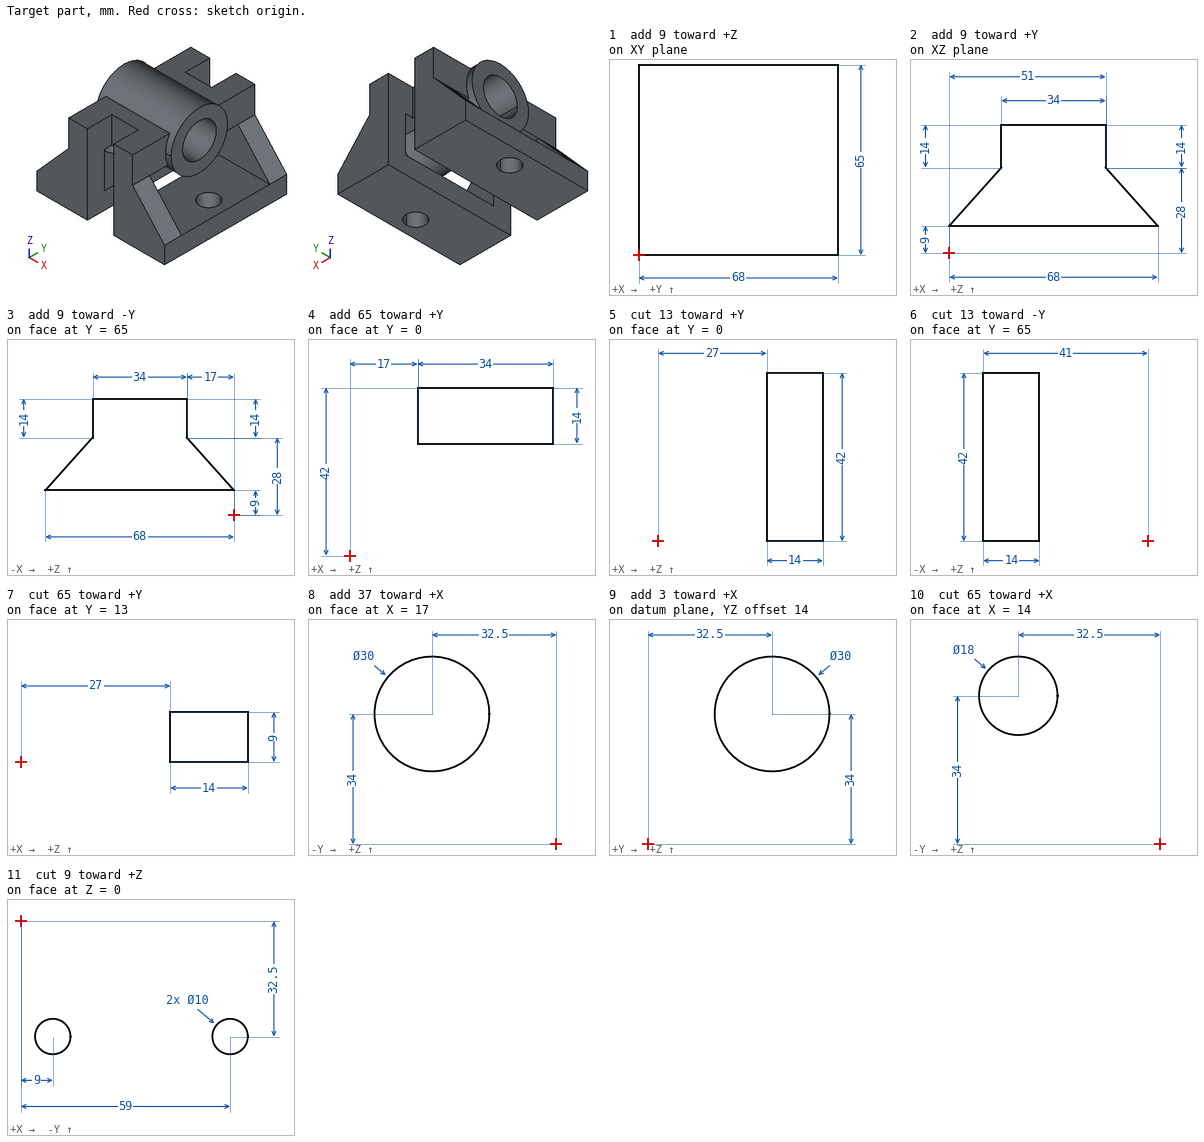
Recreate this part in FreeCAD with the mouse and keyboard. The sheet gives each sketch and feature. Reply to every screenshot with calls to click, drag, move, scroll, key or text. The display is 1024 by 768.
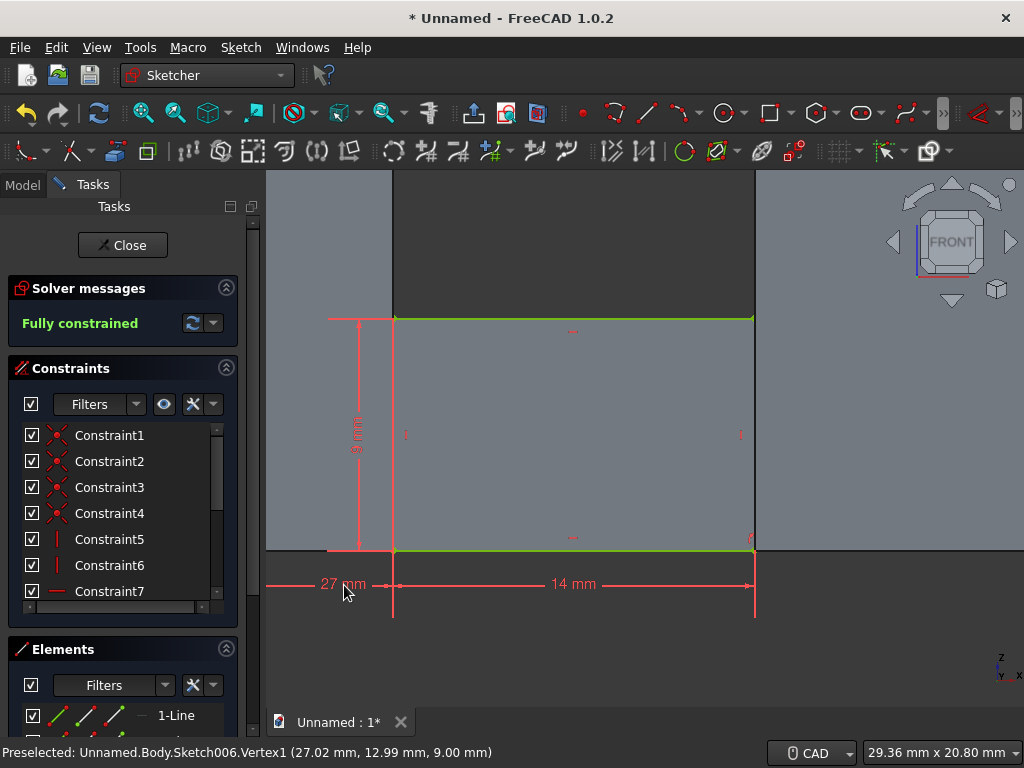
click(123, 245)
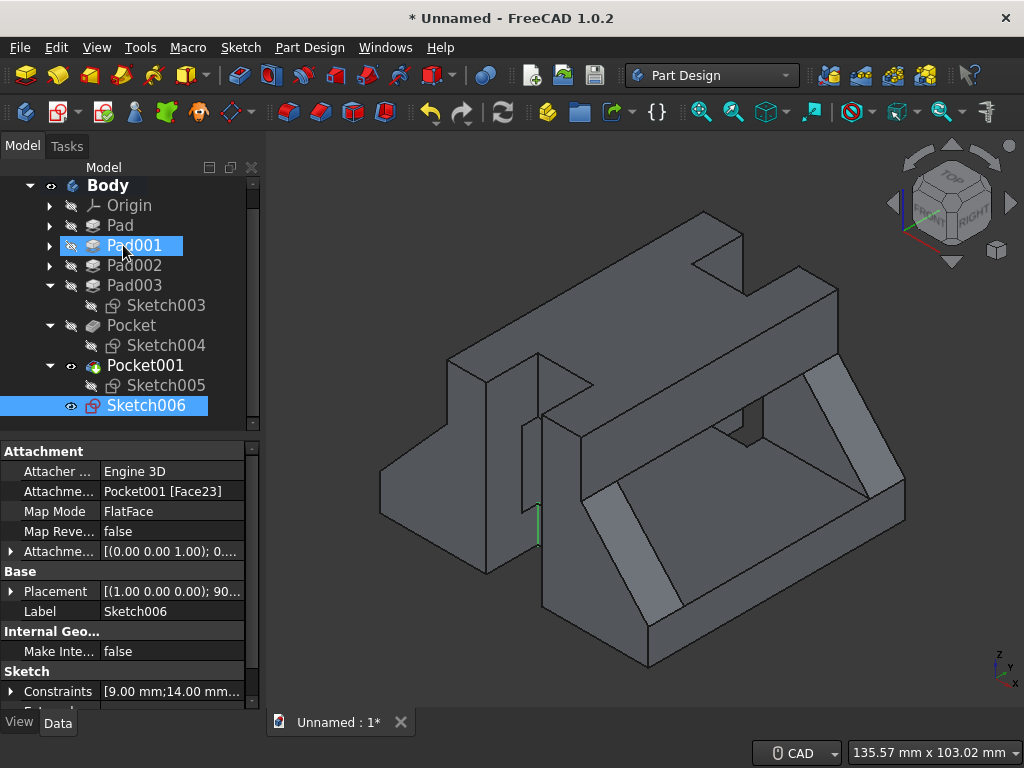
click(240, 76)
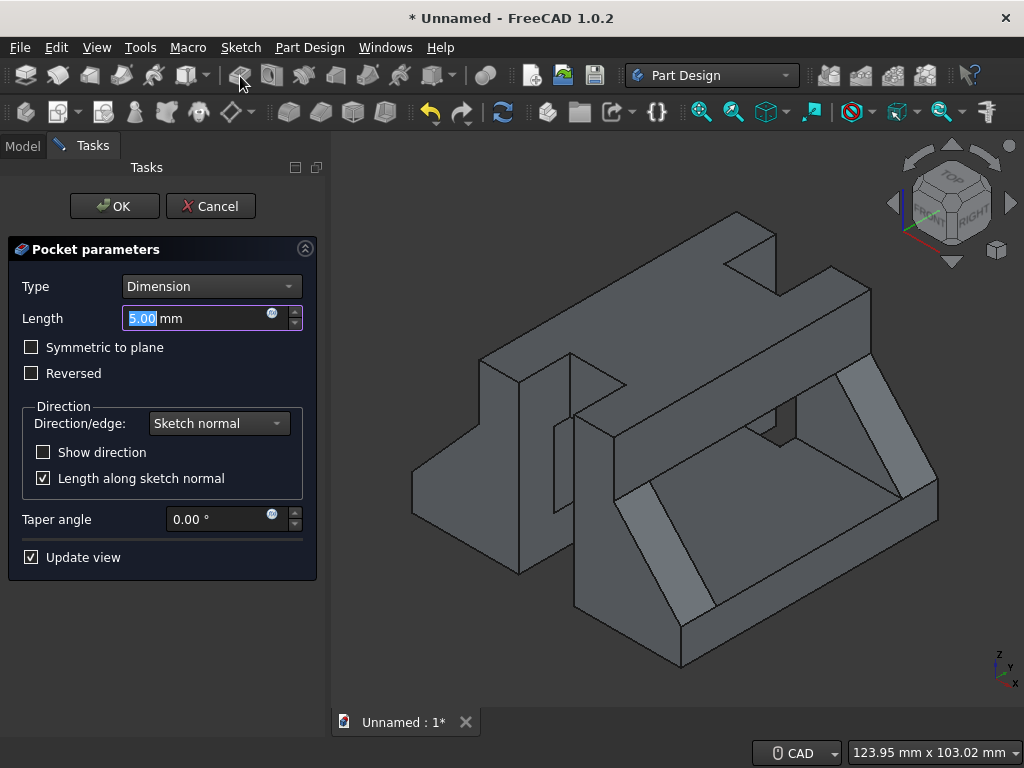
text(65)
key(Tab)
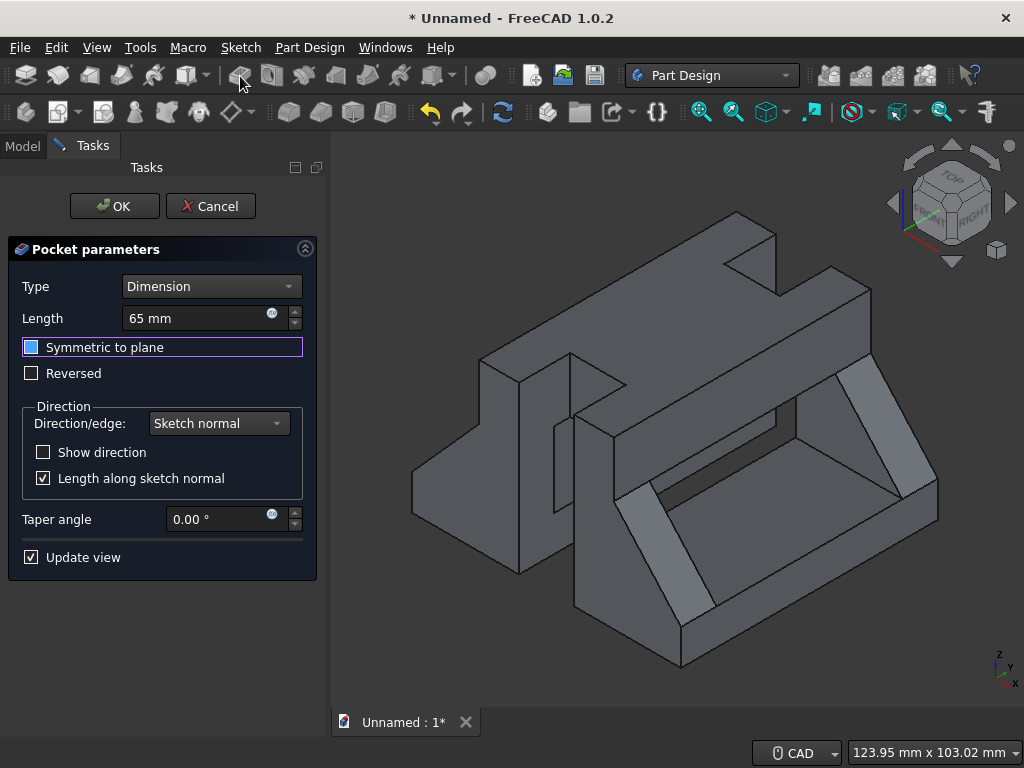
click(115, 206)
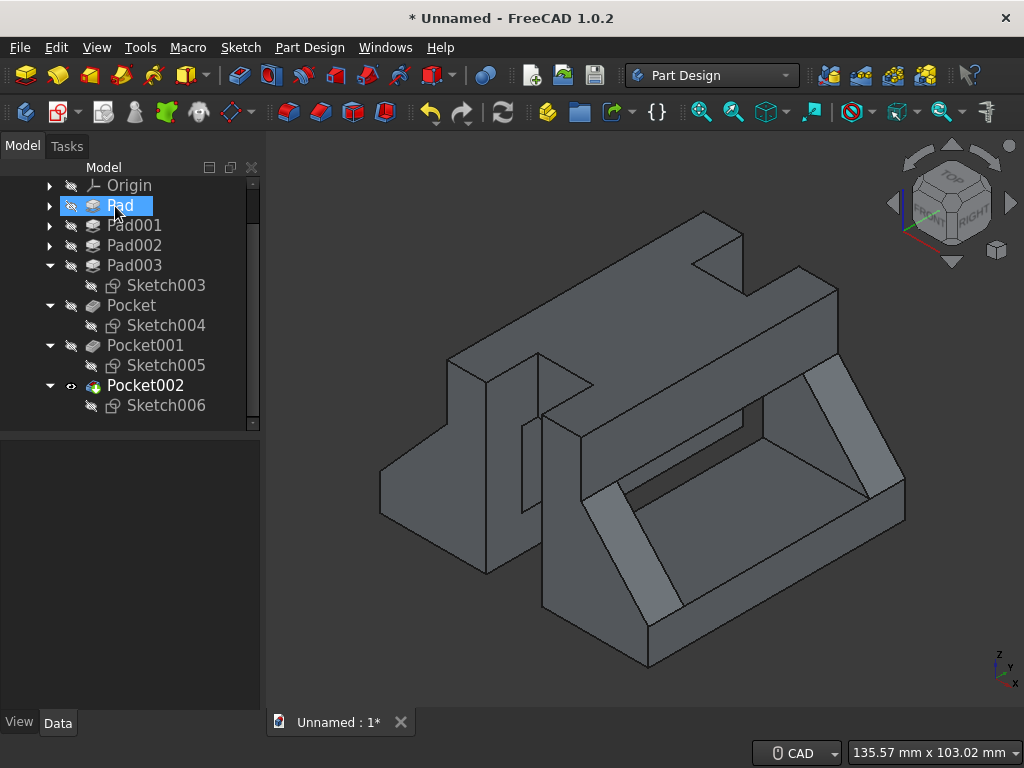
key(6)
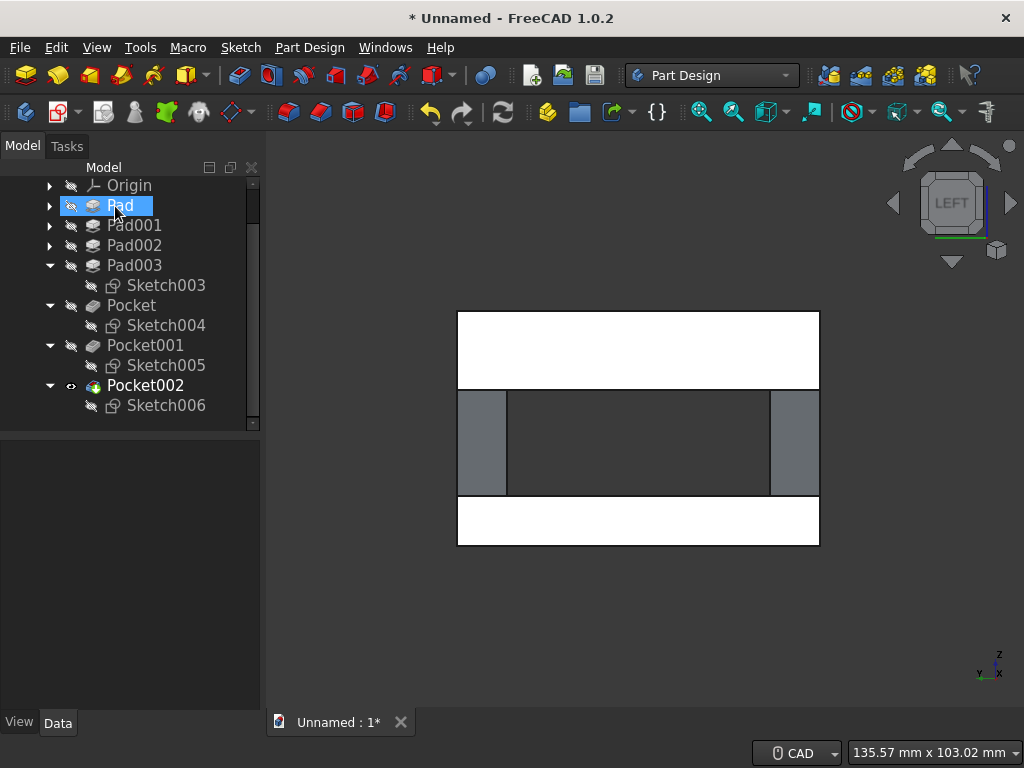
click(587, 350)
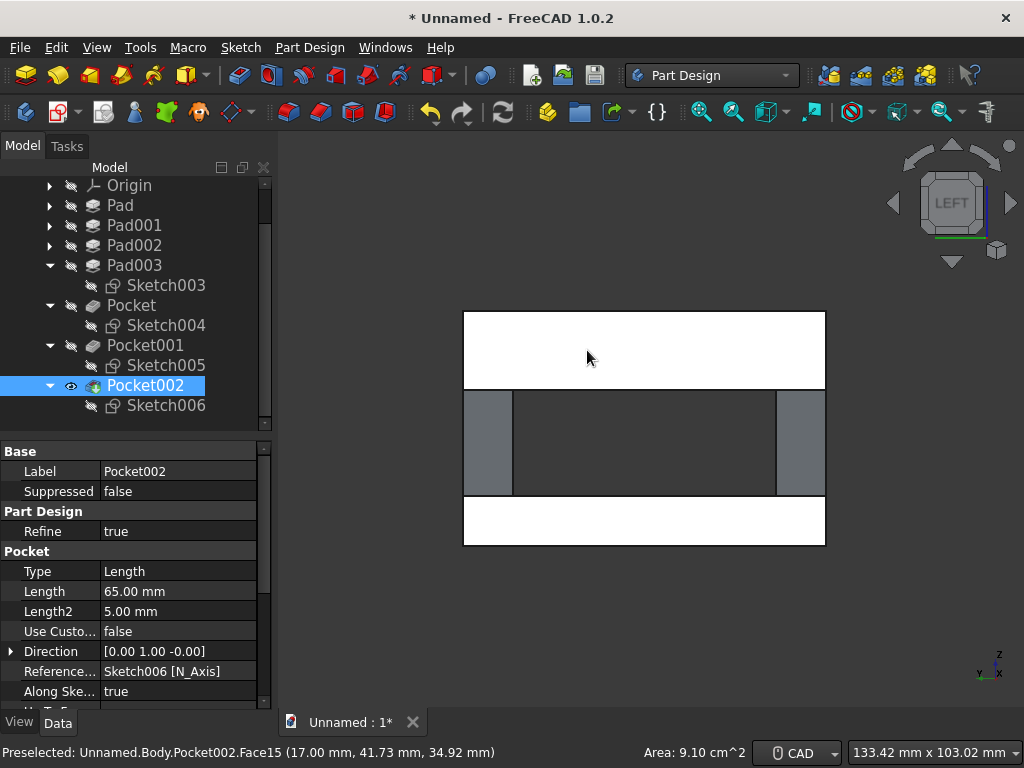
click(58, 112)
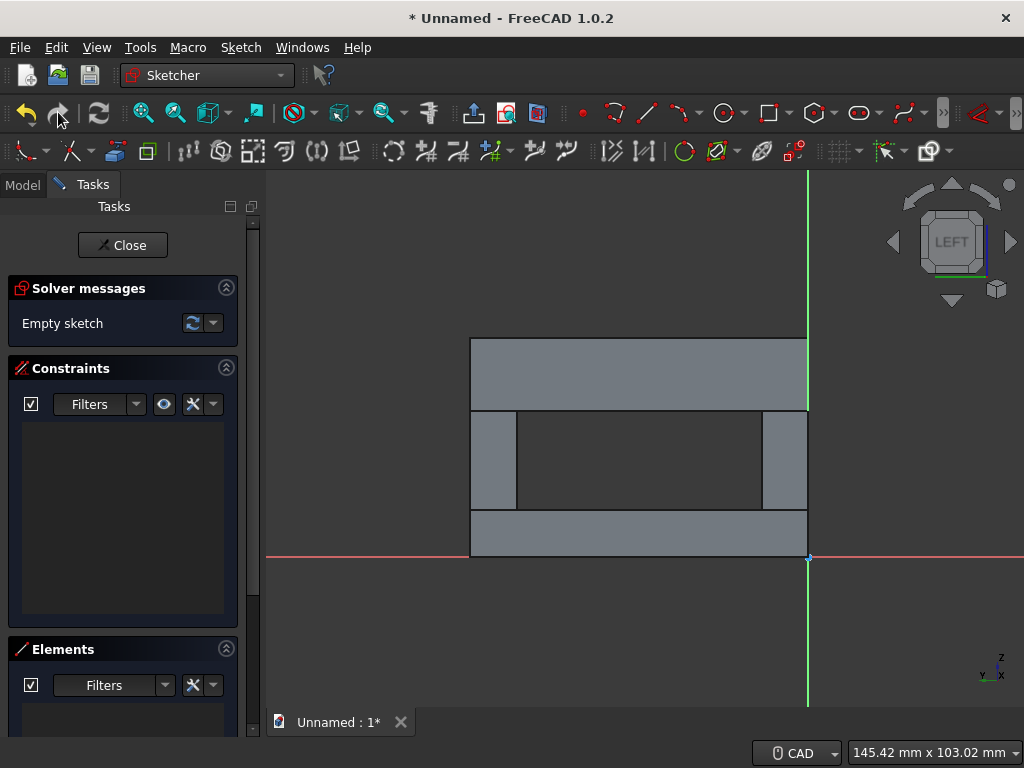
key(g)
key(c)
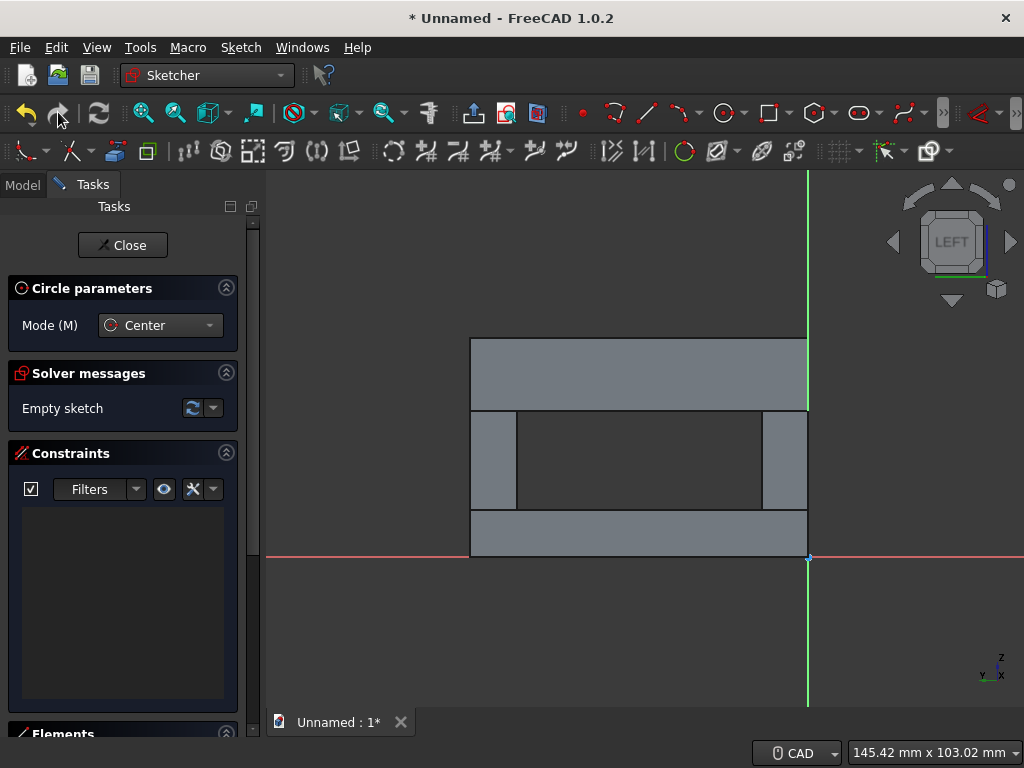
click(639, 380)
move(694, 325)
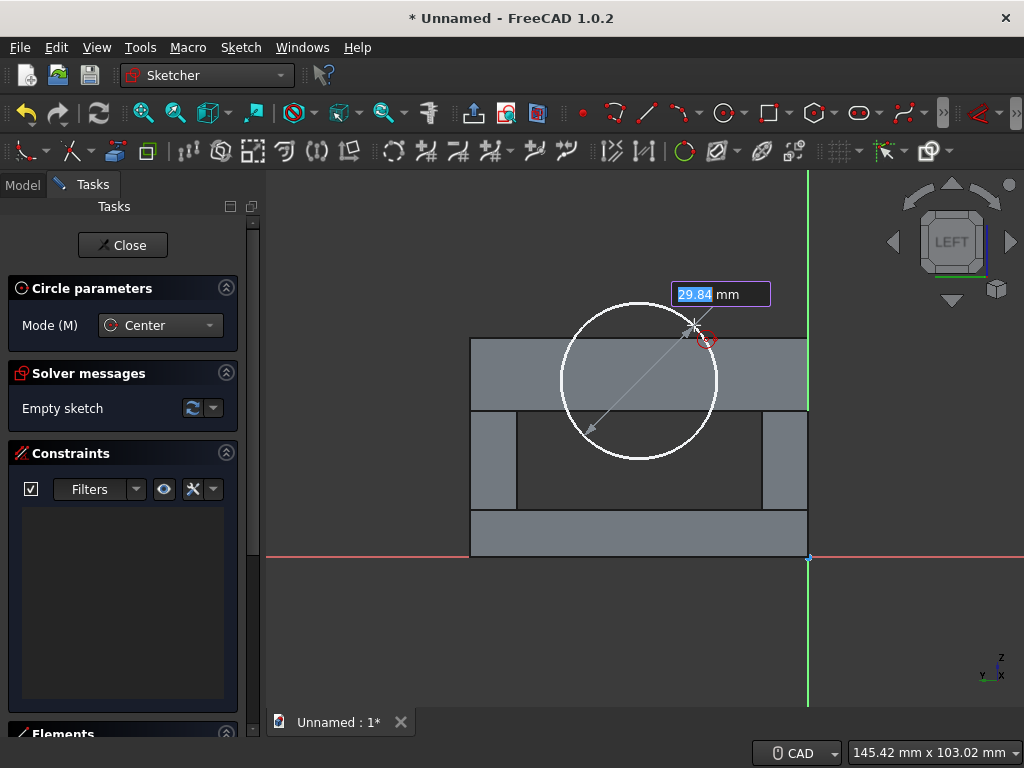
text(30)
key(Return)
key(Escape)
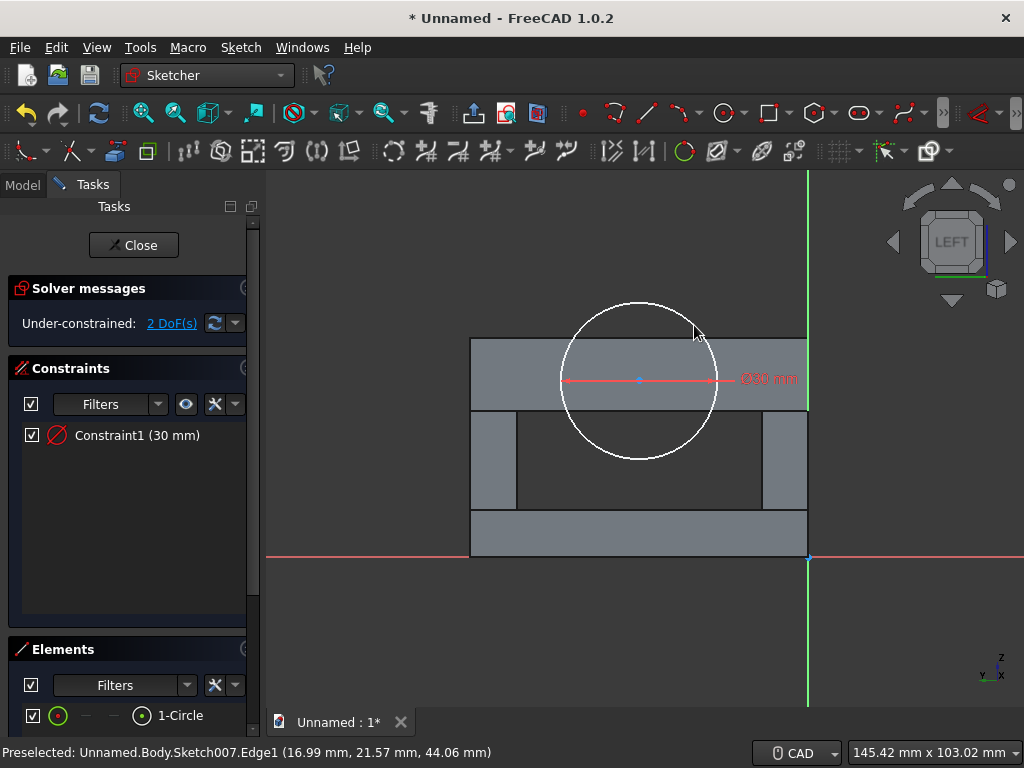
click(978, 114)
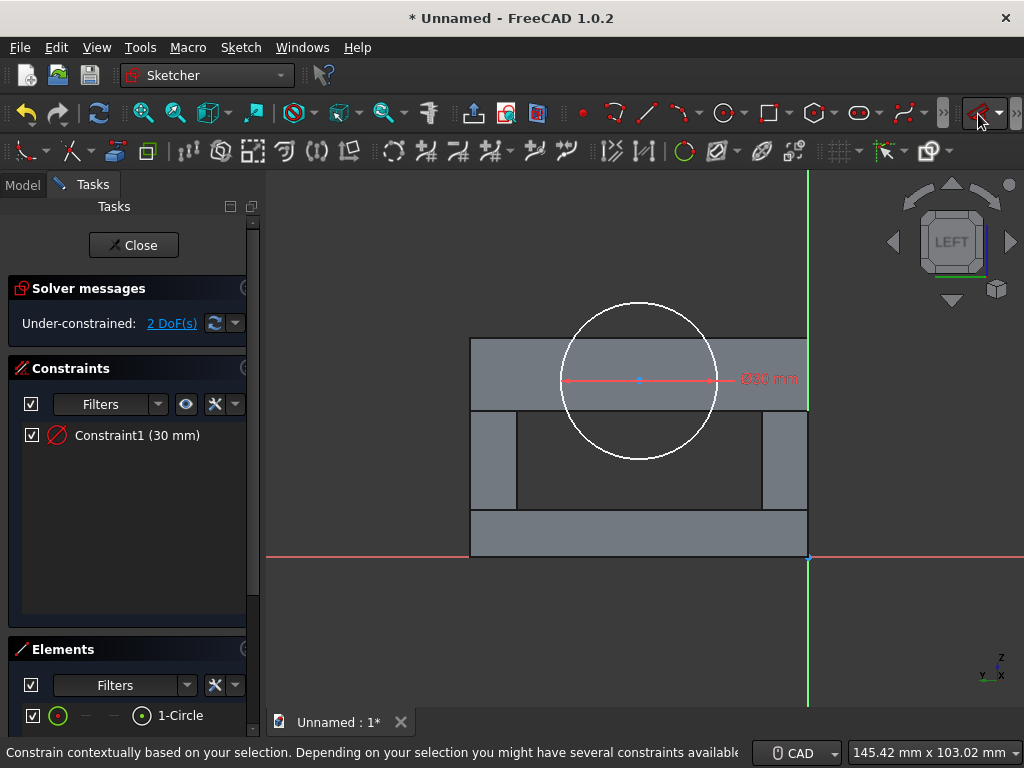
click(639, 381)
click(842, 469)